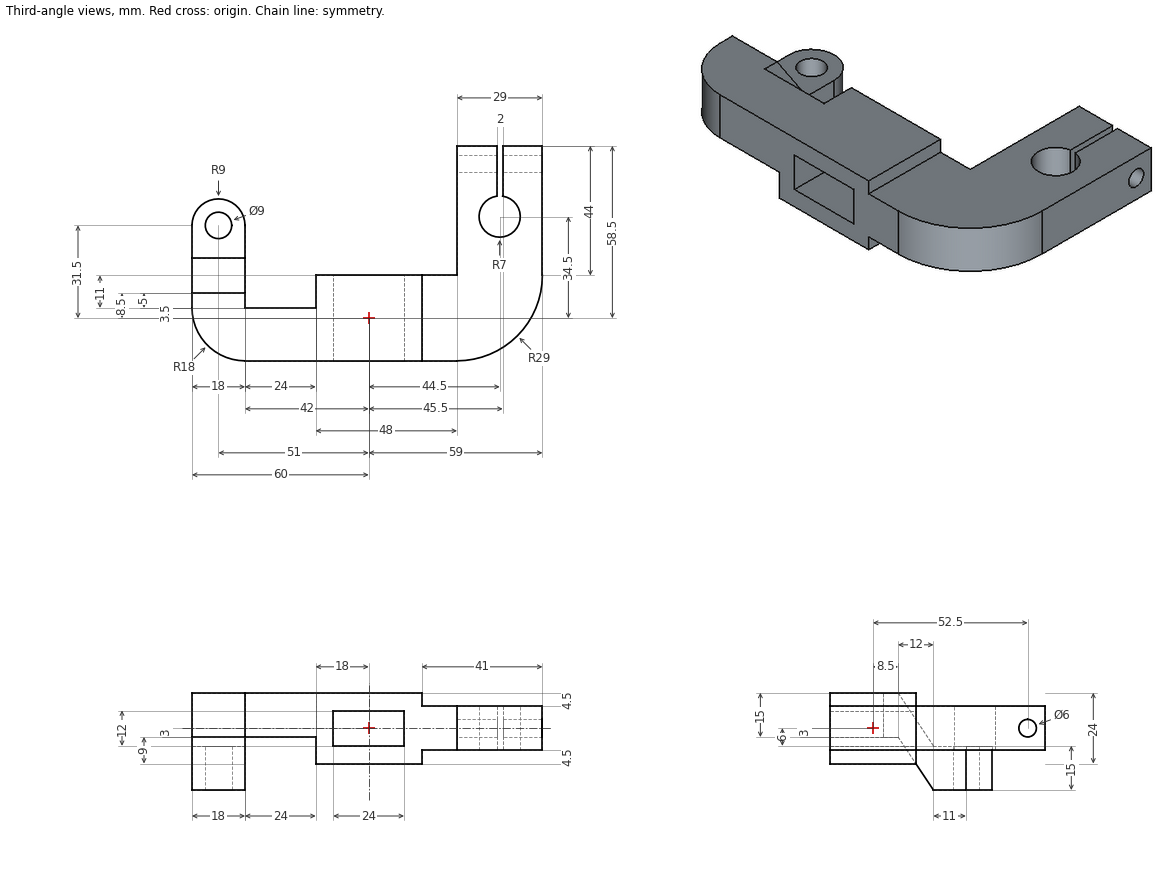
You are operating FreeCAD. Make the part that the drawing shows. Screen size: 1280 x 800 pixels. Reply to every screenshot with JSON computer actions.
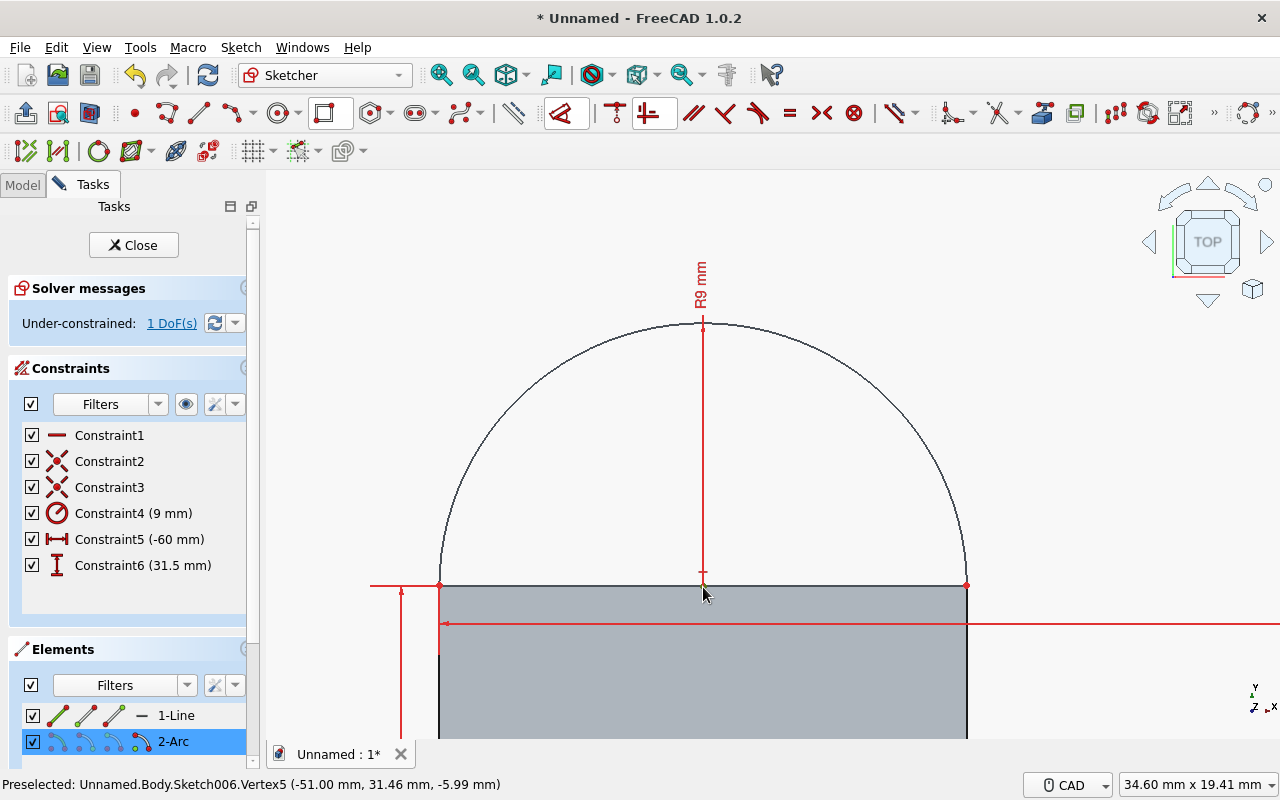
{"action": "left_click", "coordinate": [584, 114]}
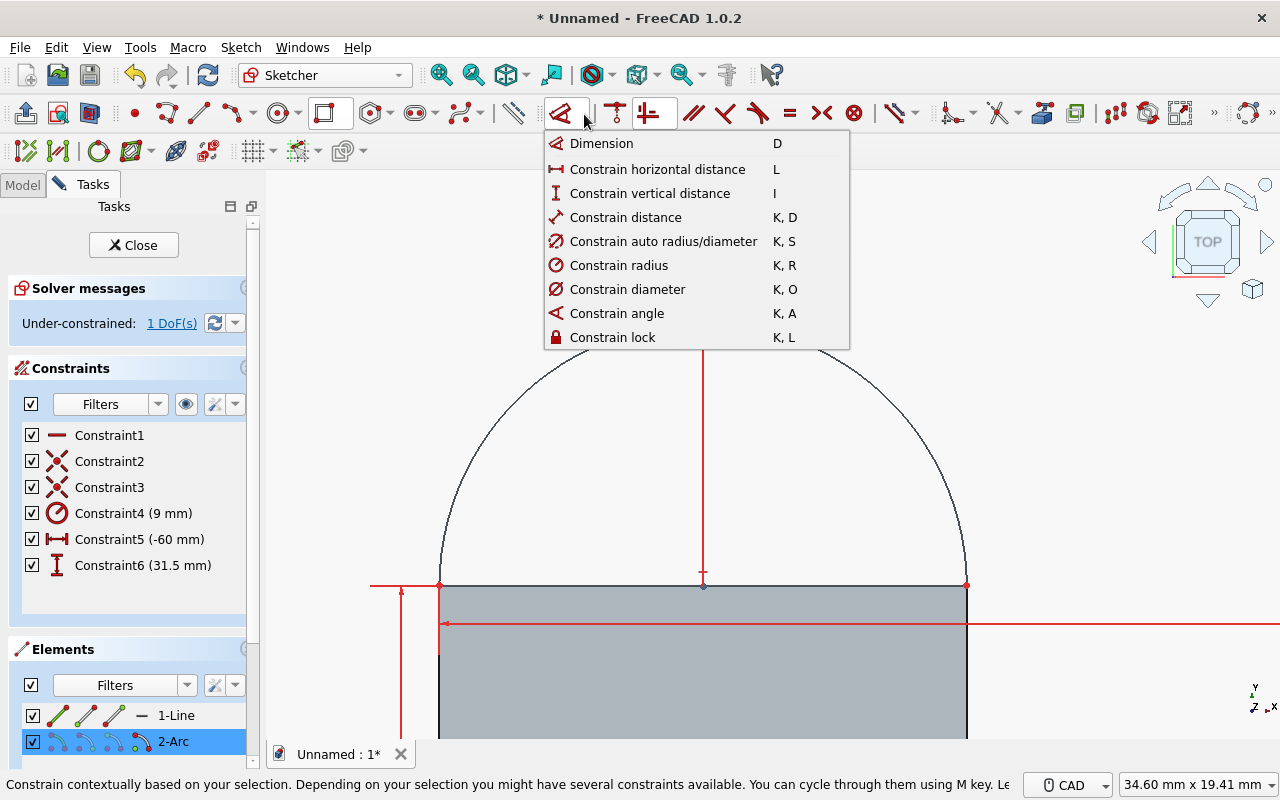
{"action": "left_click", "coordinate": [697, 193]}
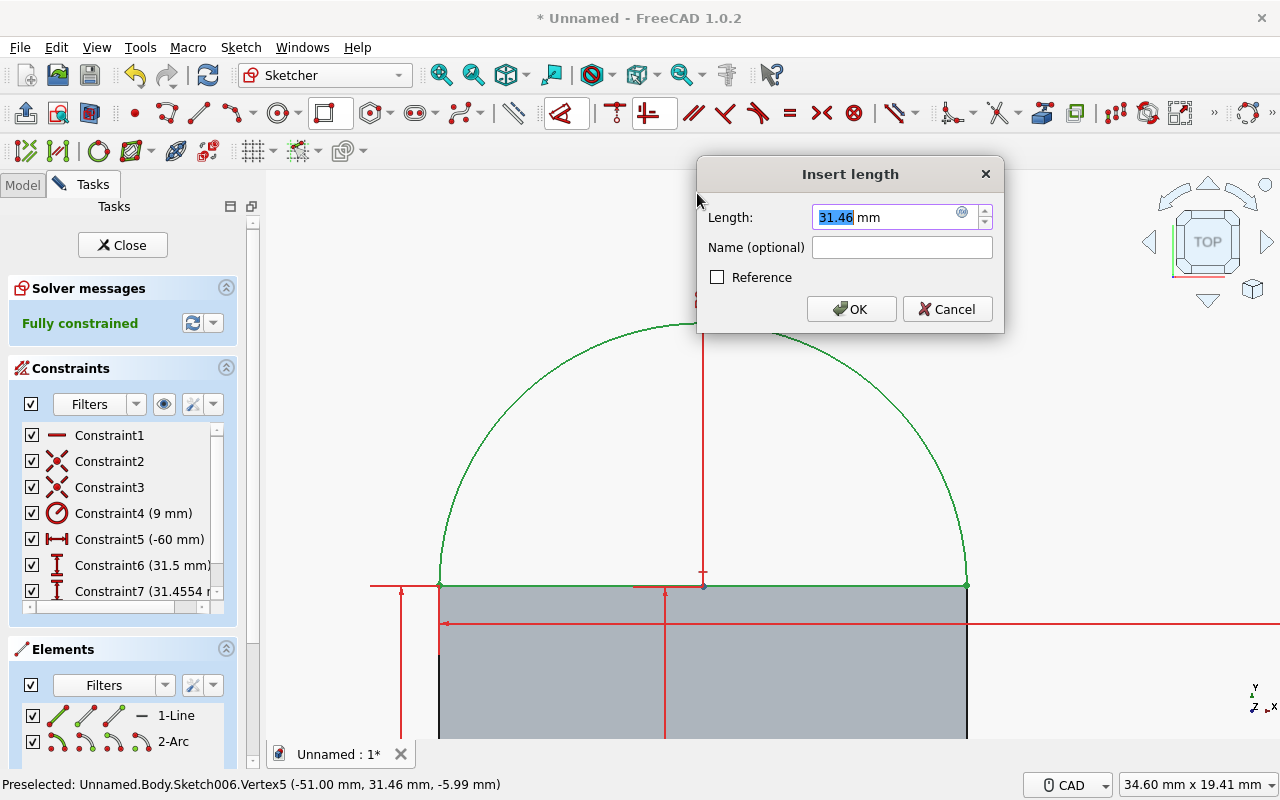
{"action": "type", "text": "31.5"}
{"action": "key", "text": "Return"}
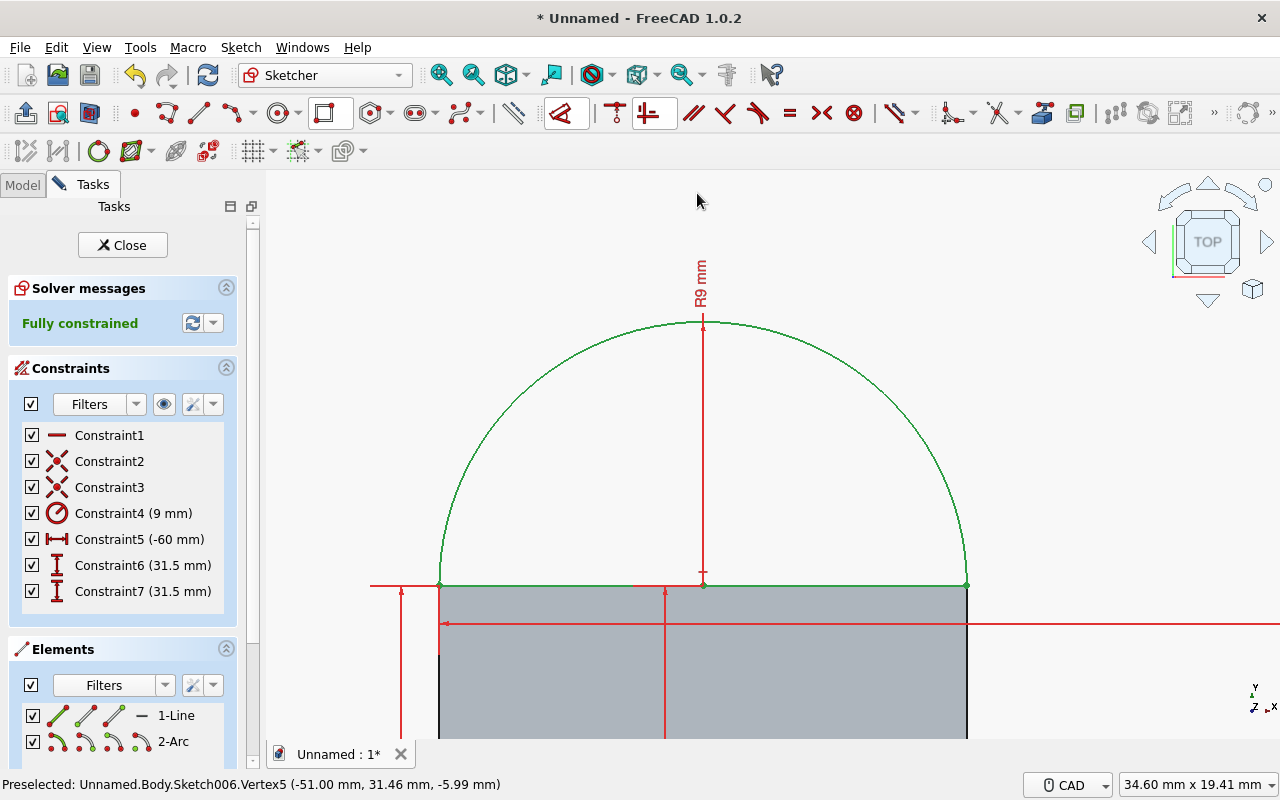
{"action": "left_click", "coordinate": [123, 245]}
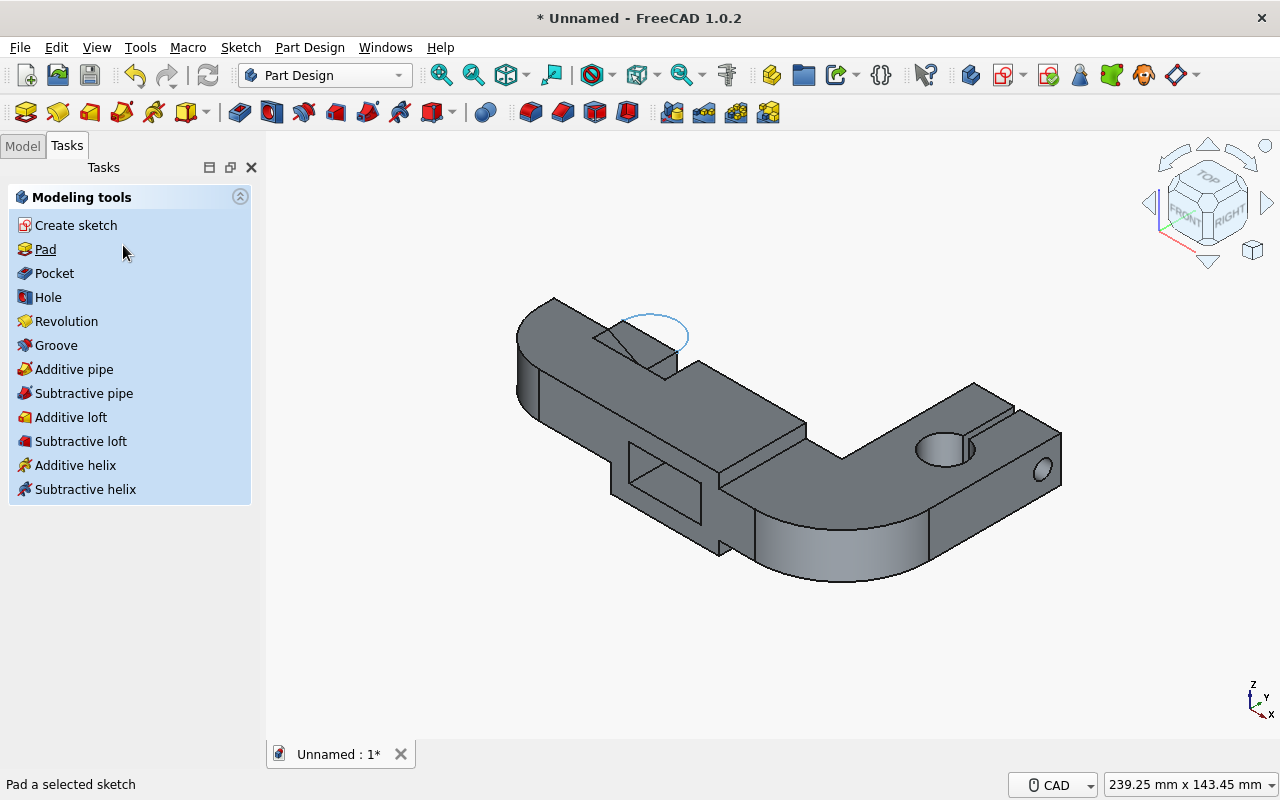
{"action": "left_click", "coordinate": [26, 112]}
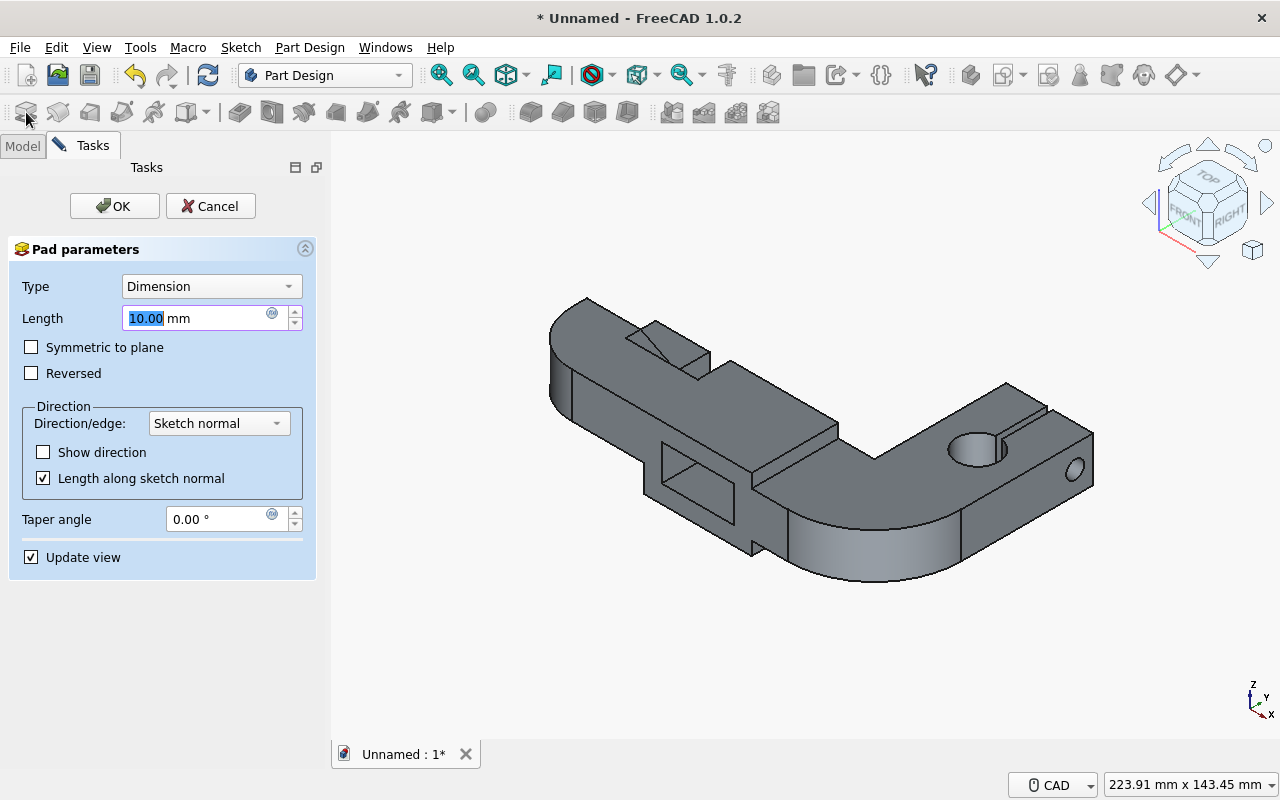
{"action": "type", "text": "15"}
{"action": "key", "text": "Tab"}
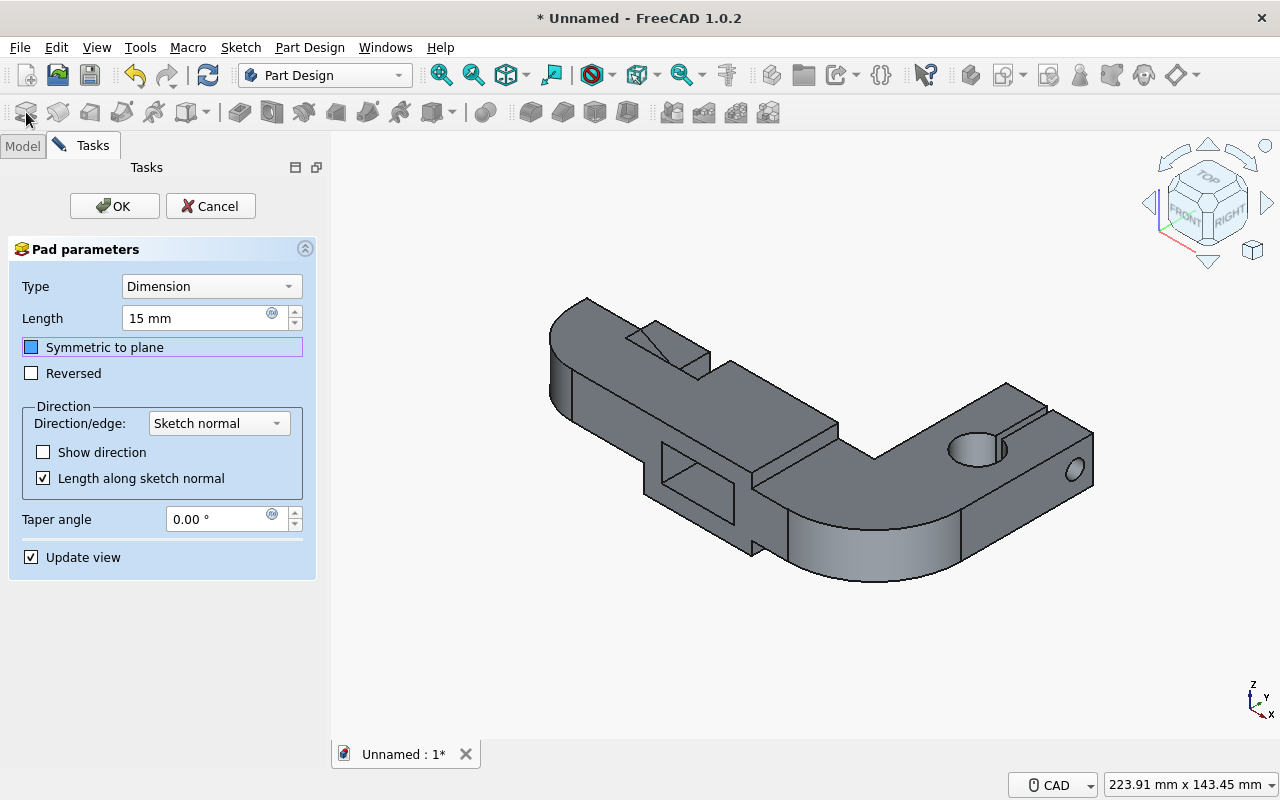
{"action": "left_click", "coordinate": [30, 373]}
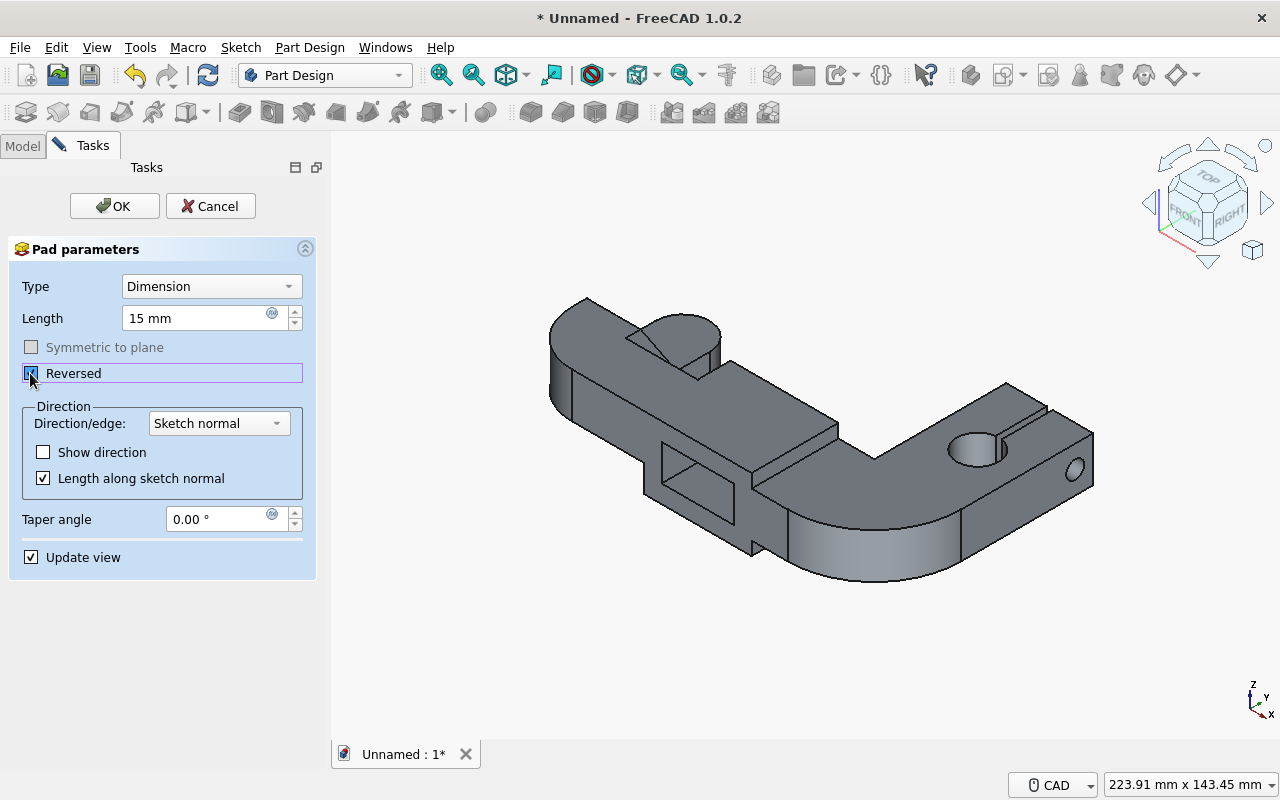
{"action": "left_click", "coordinate": [115, 206]}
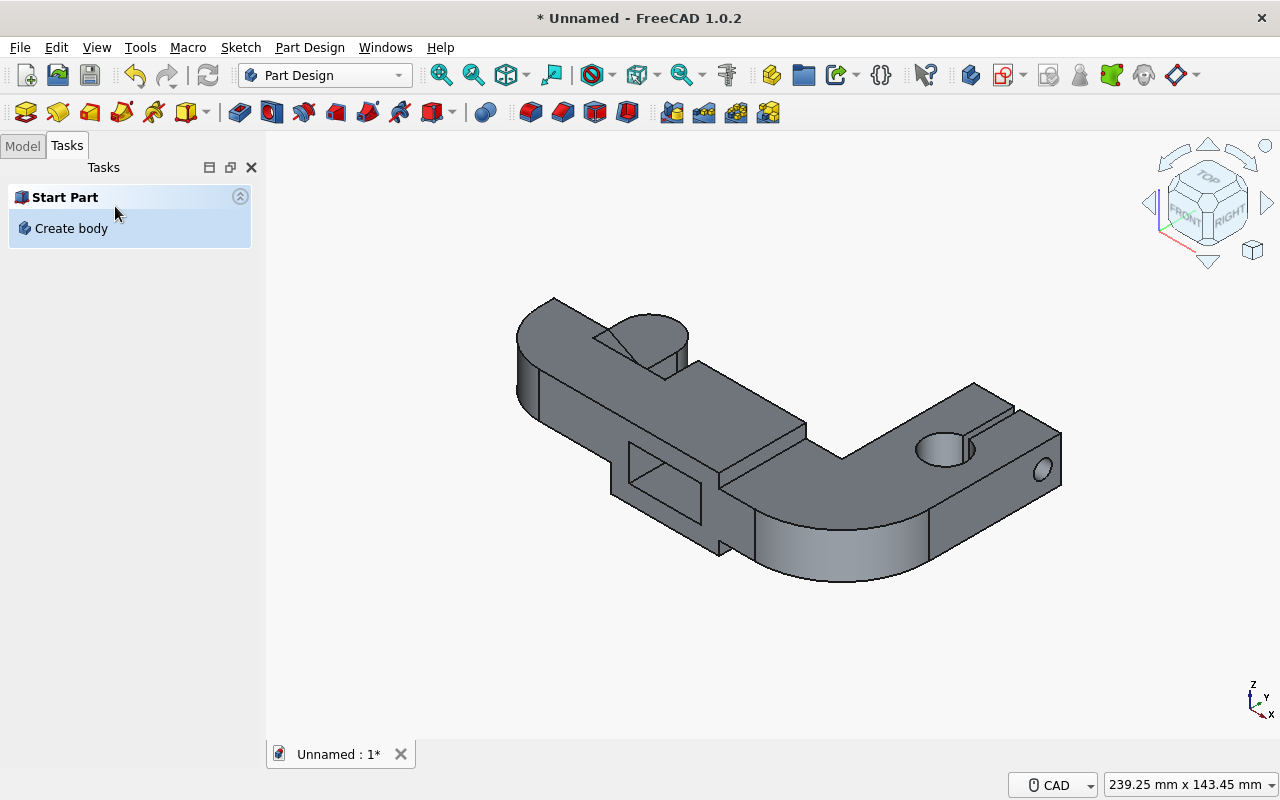
{"action": "left_click", "coordinate": [647, 337]}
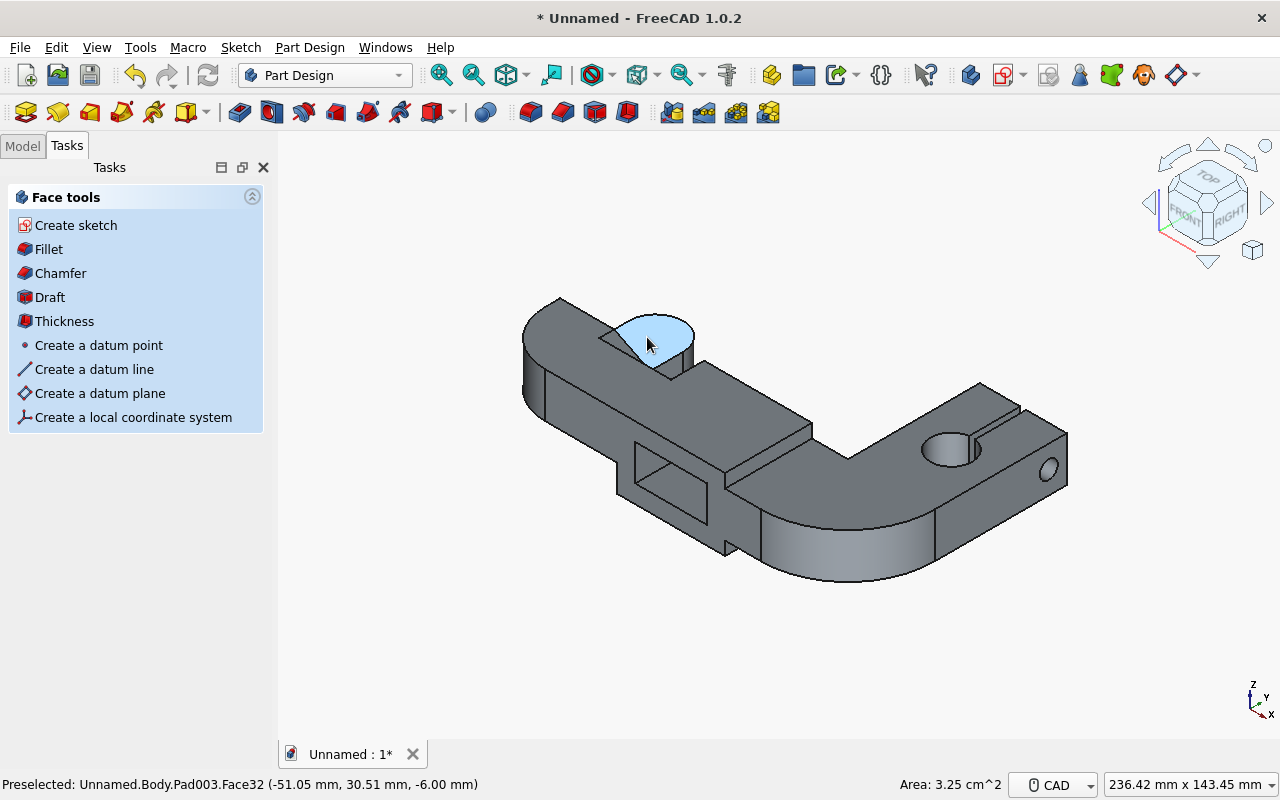
{"action": "left_click", "coordinate": [1004, 76]}